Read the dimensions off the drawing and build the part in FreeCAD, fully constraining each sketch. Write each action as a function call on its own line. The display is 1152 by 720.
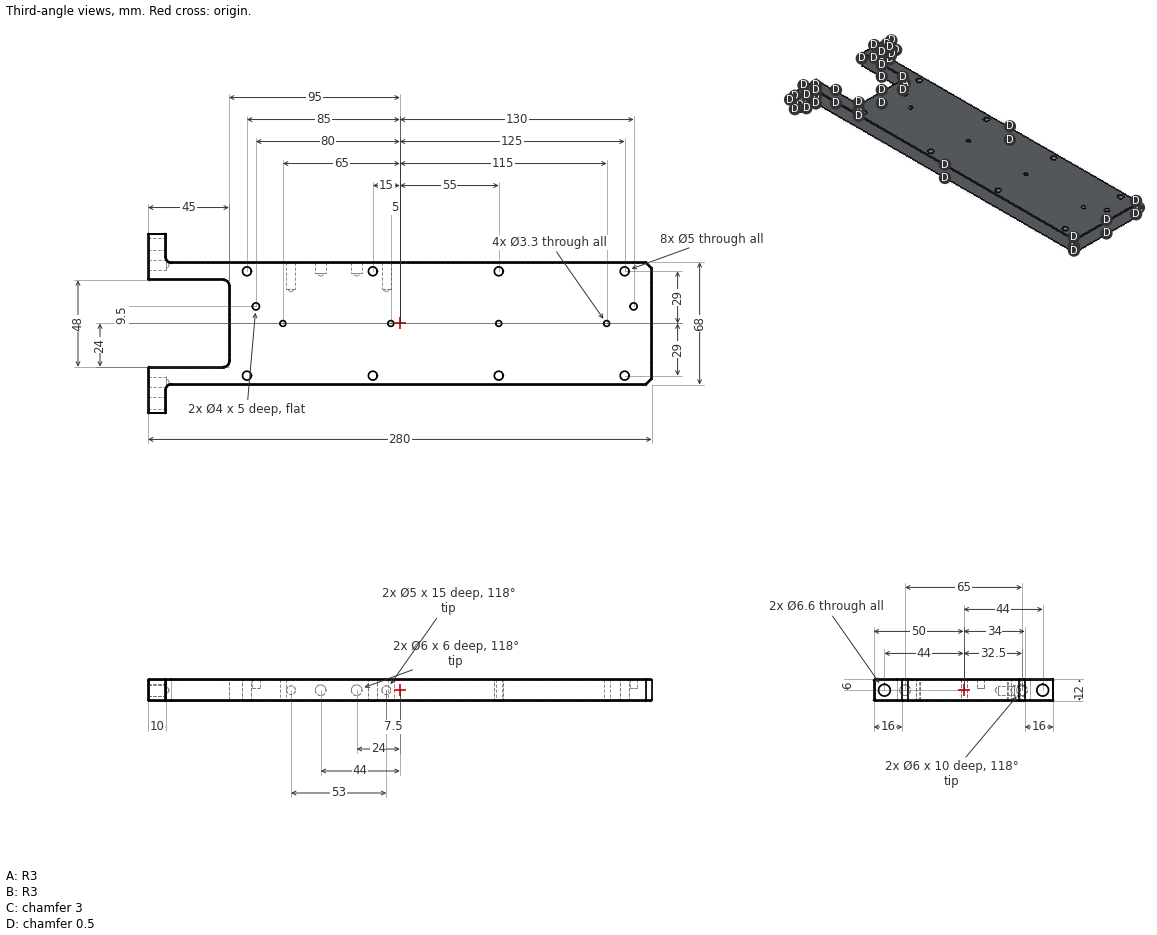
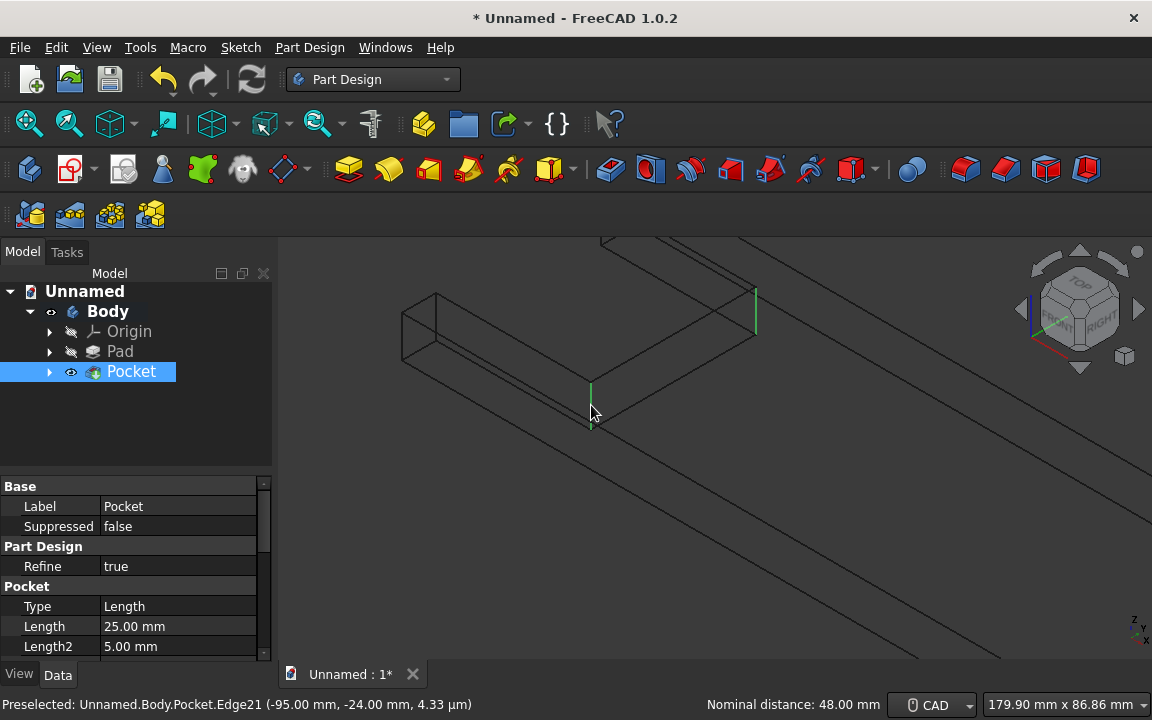
key(v)
key(1)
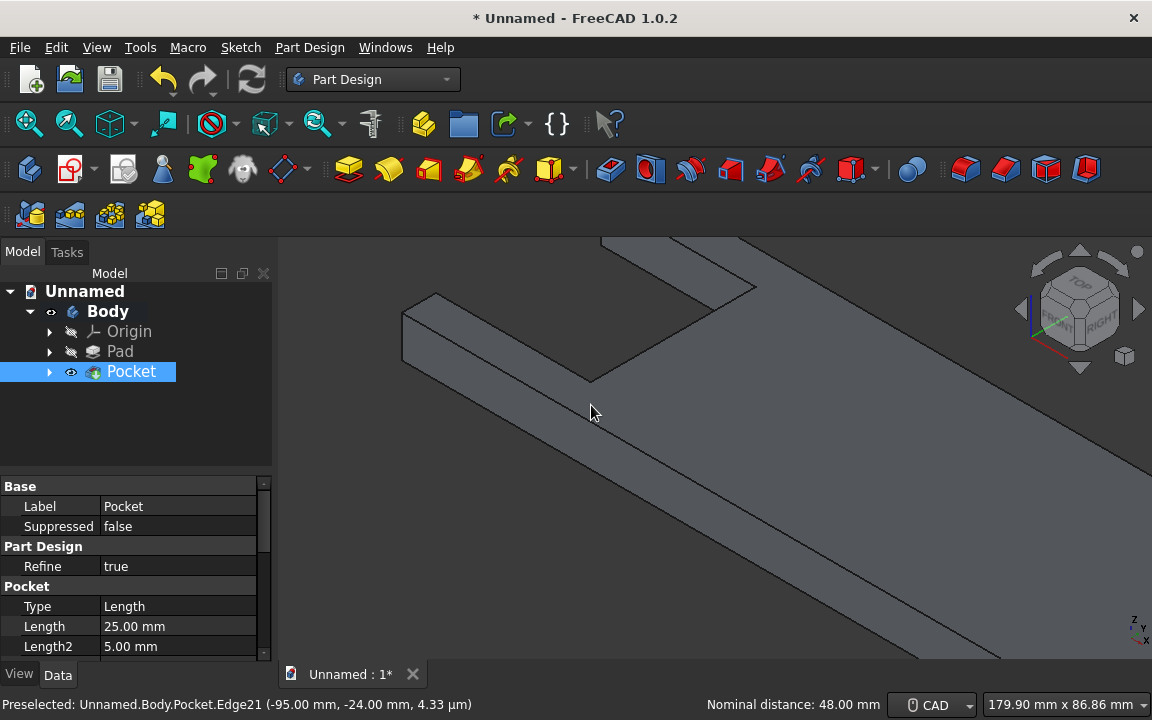
click(966, 170)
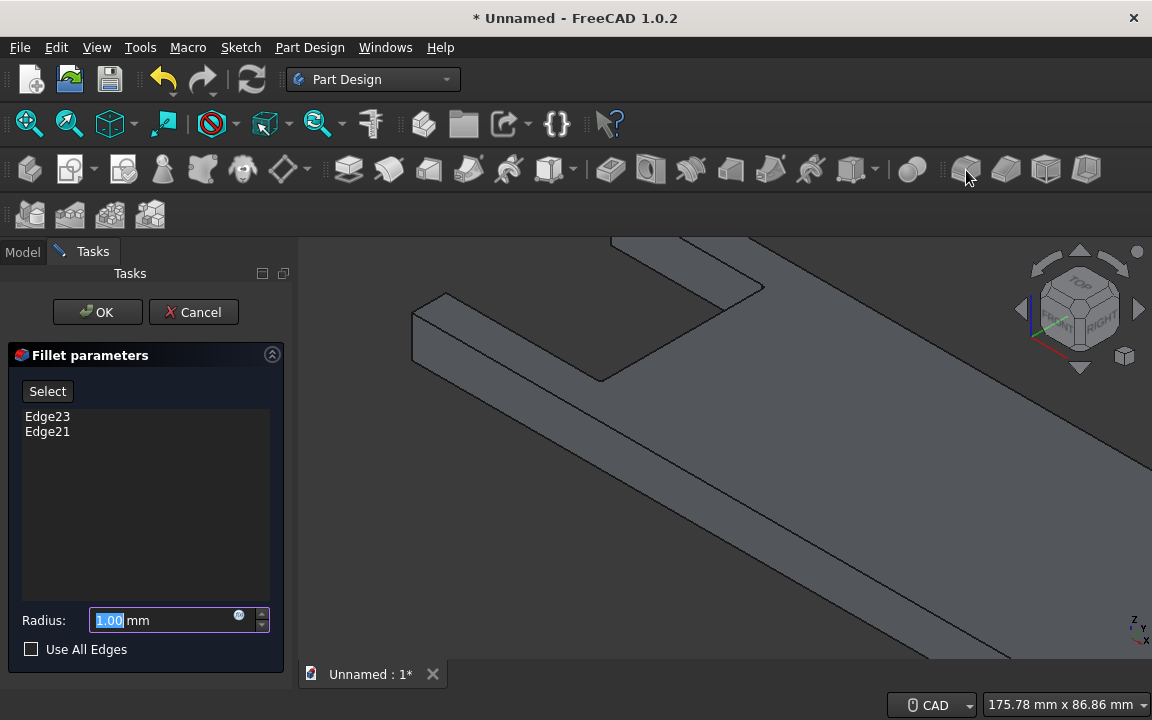
text(3)
key(Tab)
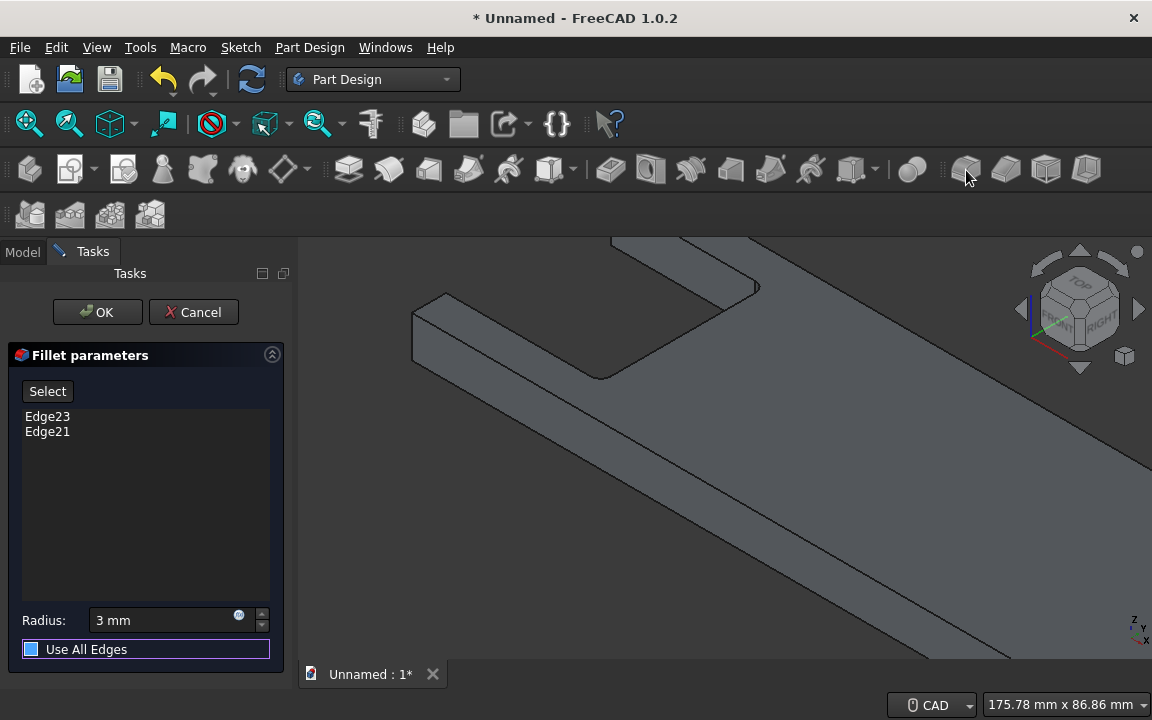
click(98, 312)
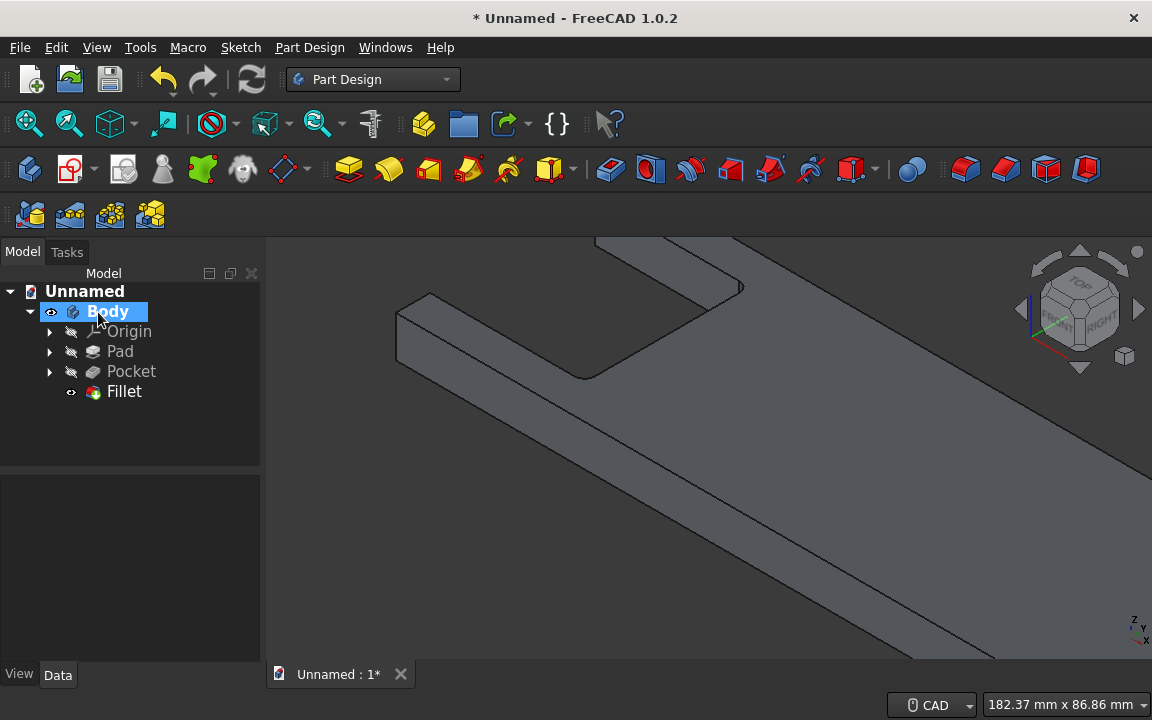
click(30, 124)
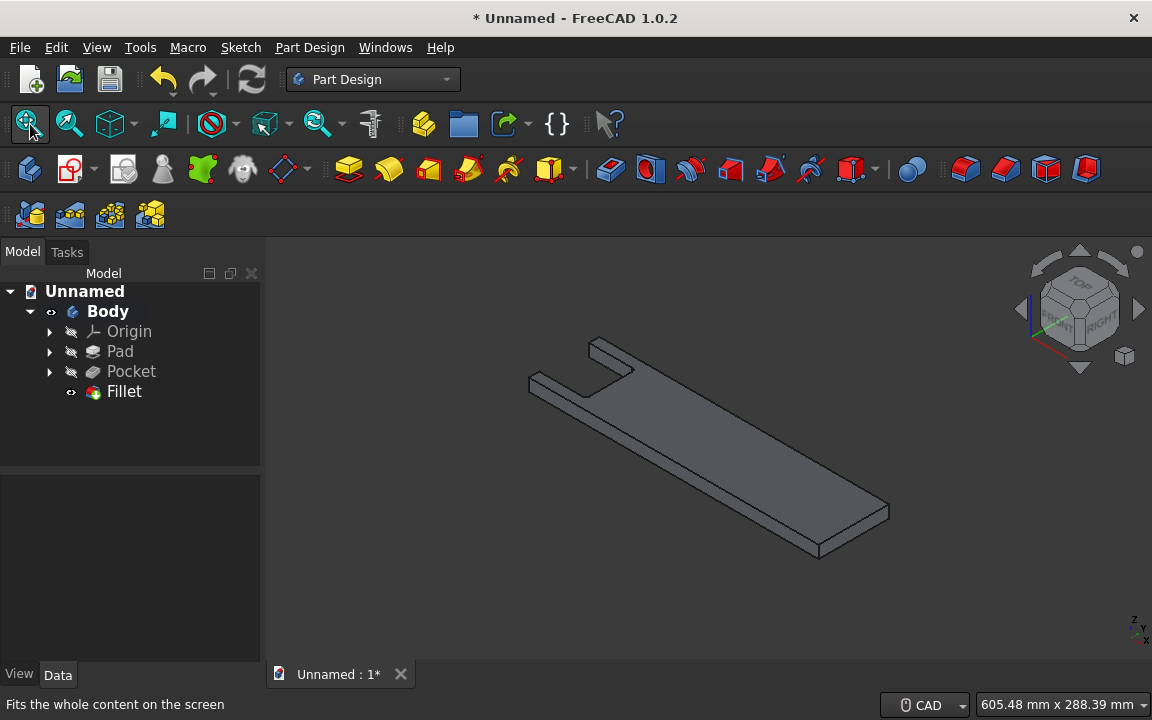
key(6)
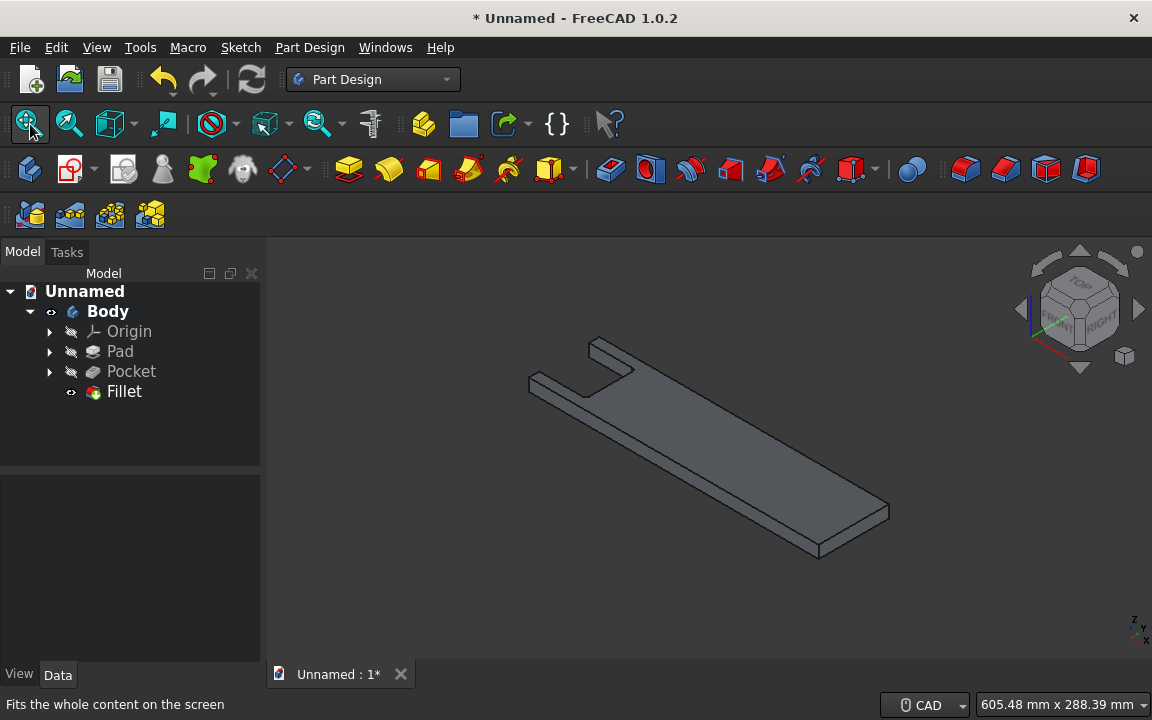
click(30, 124)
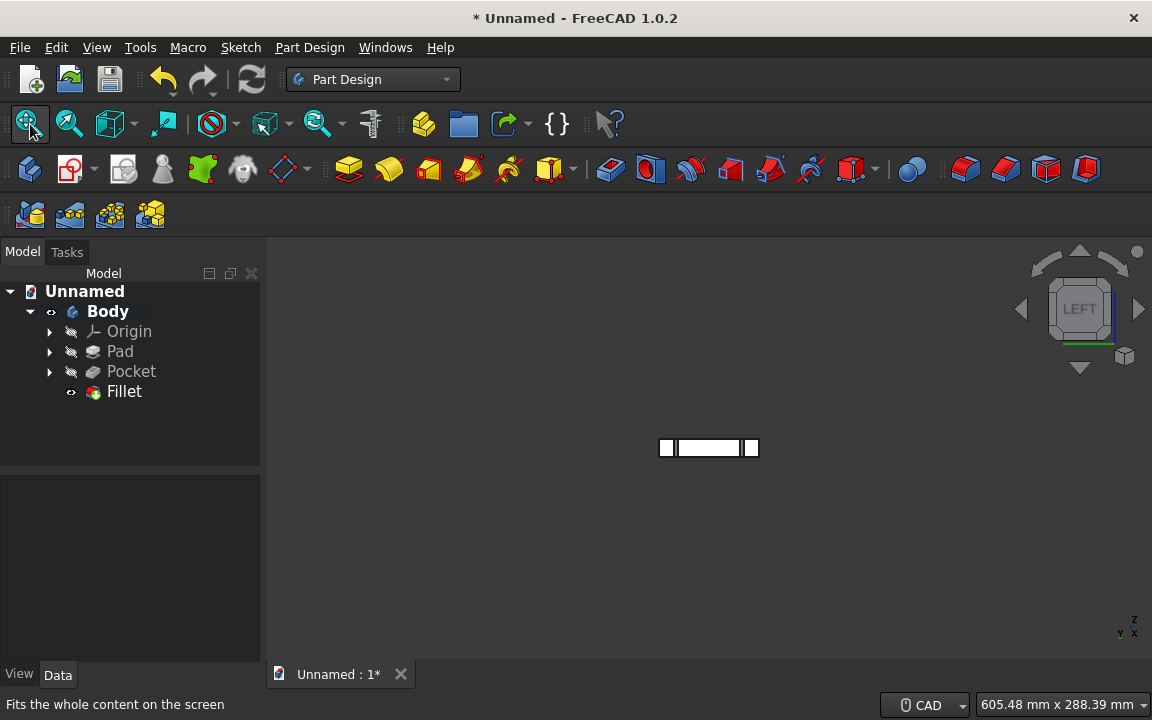
key(2)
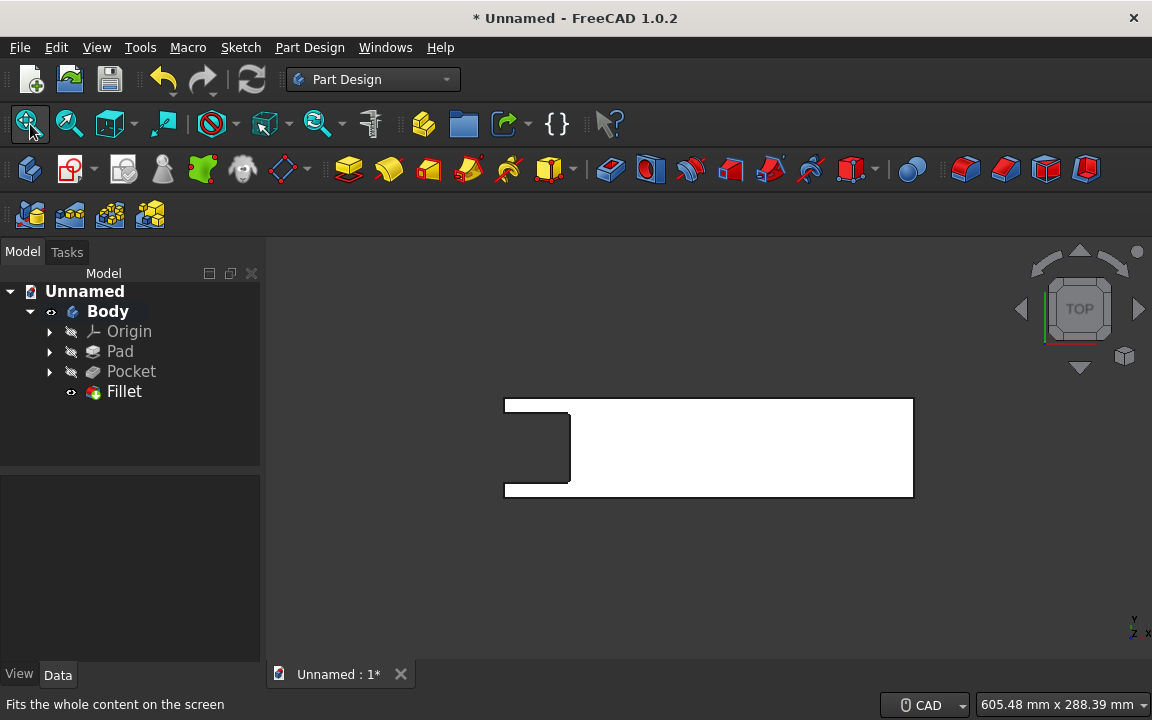
key(1)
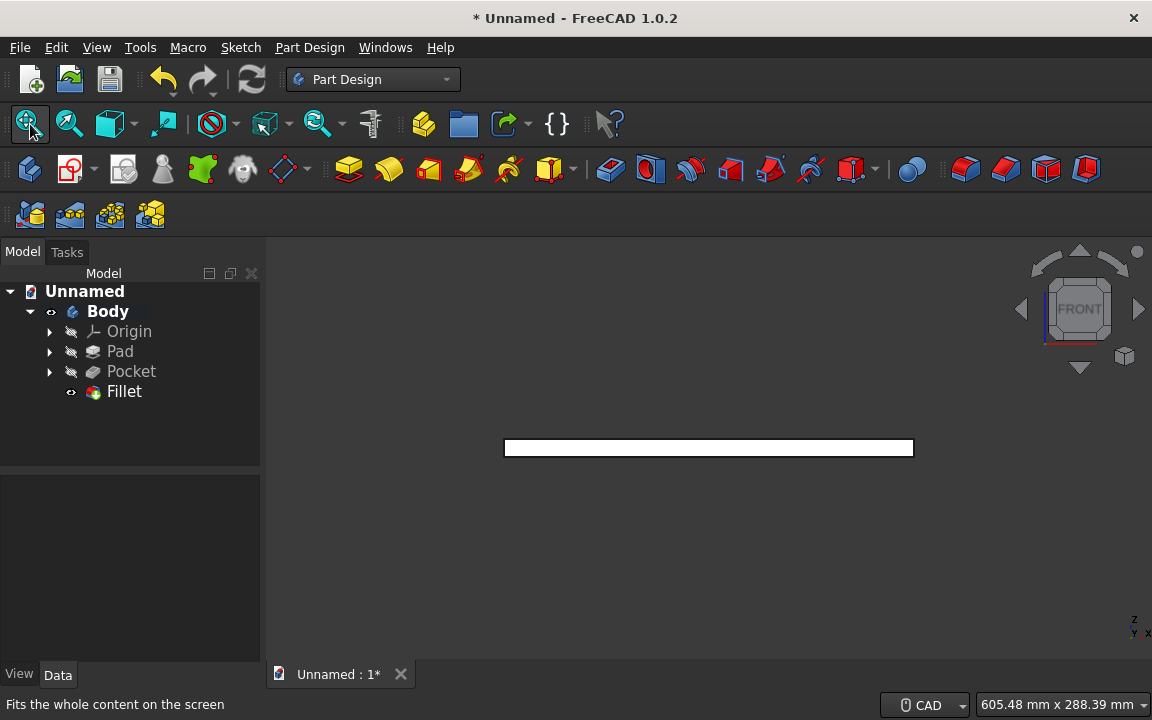
click(50, 332)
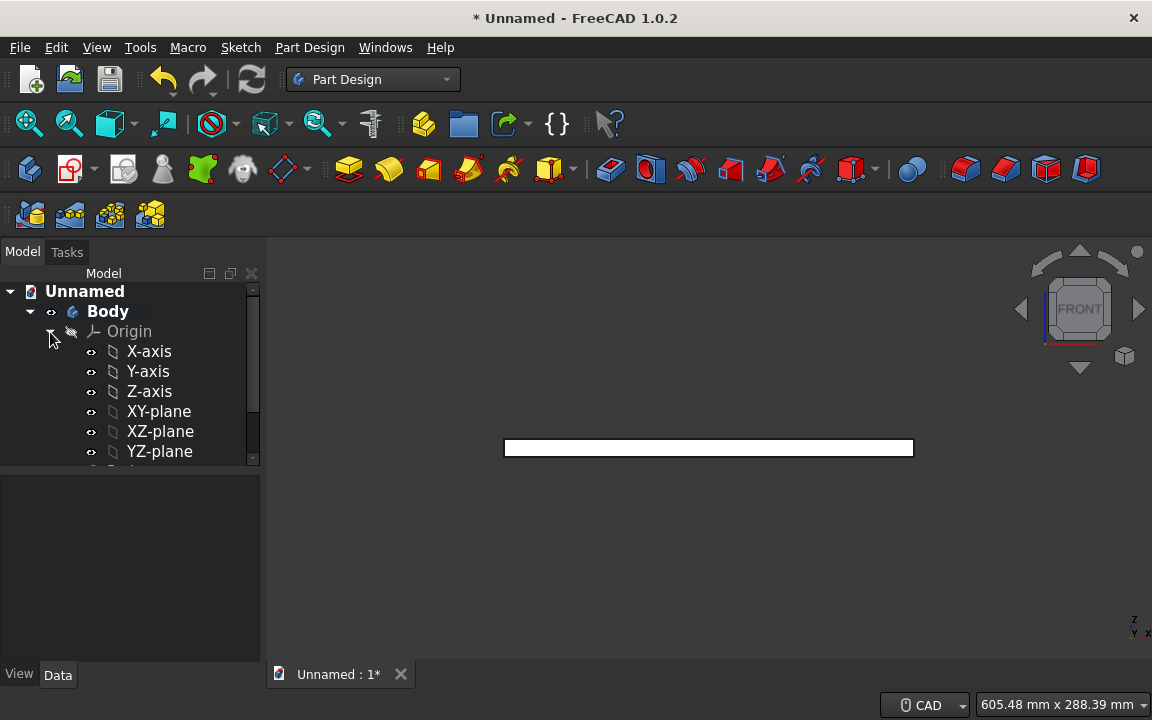
click(136, 452)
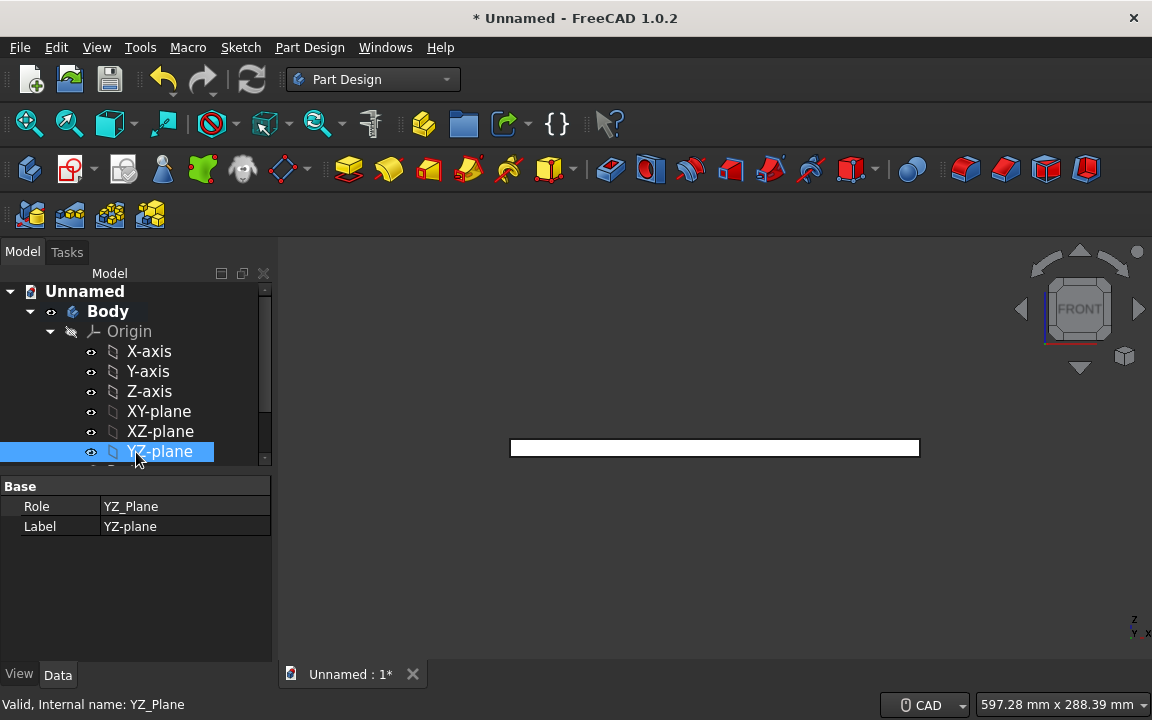
click(284, 170)